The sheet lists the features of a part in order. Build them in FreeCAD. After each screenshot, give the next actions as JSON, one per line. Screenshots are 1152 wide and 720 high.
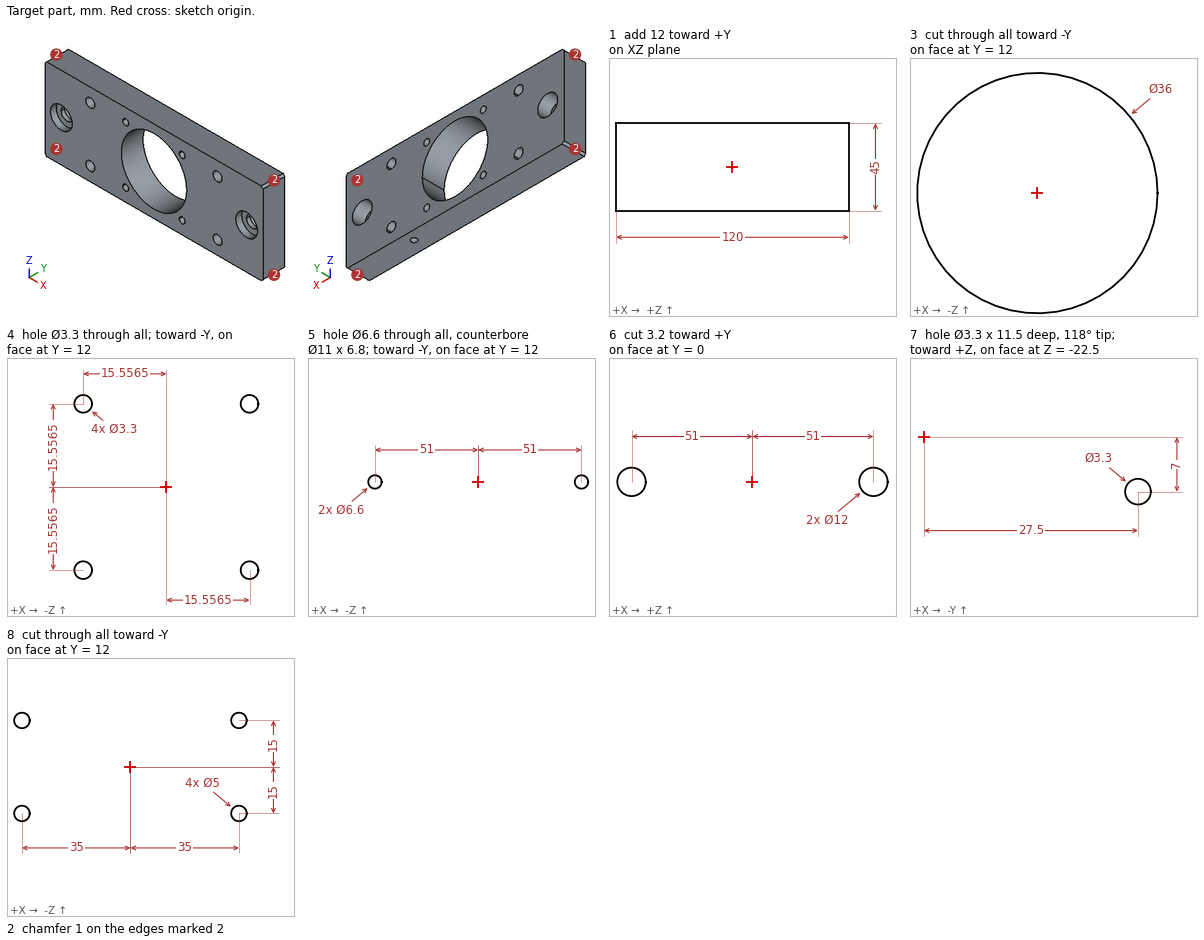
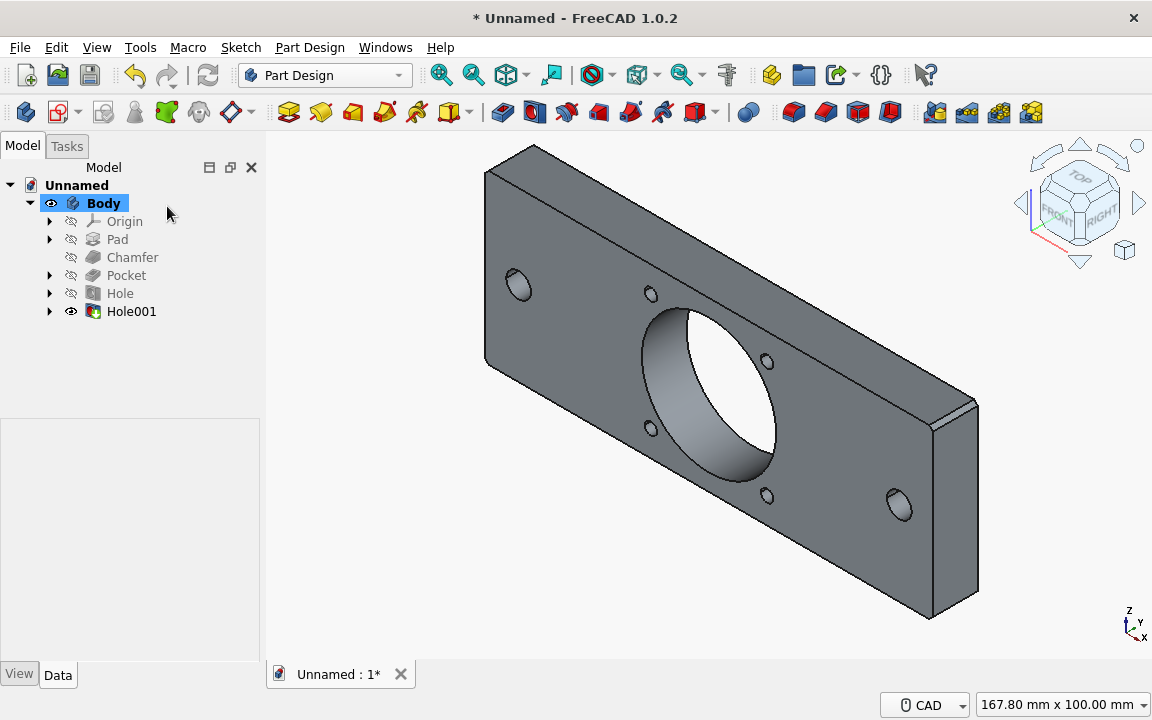
{"action": "left_click", "coordinate": [581, 292]}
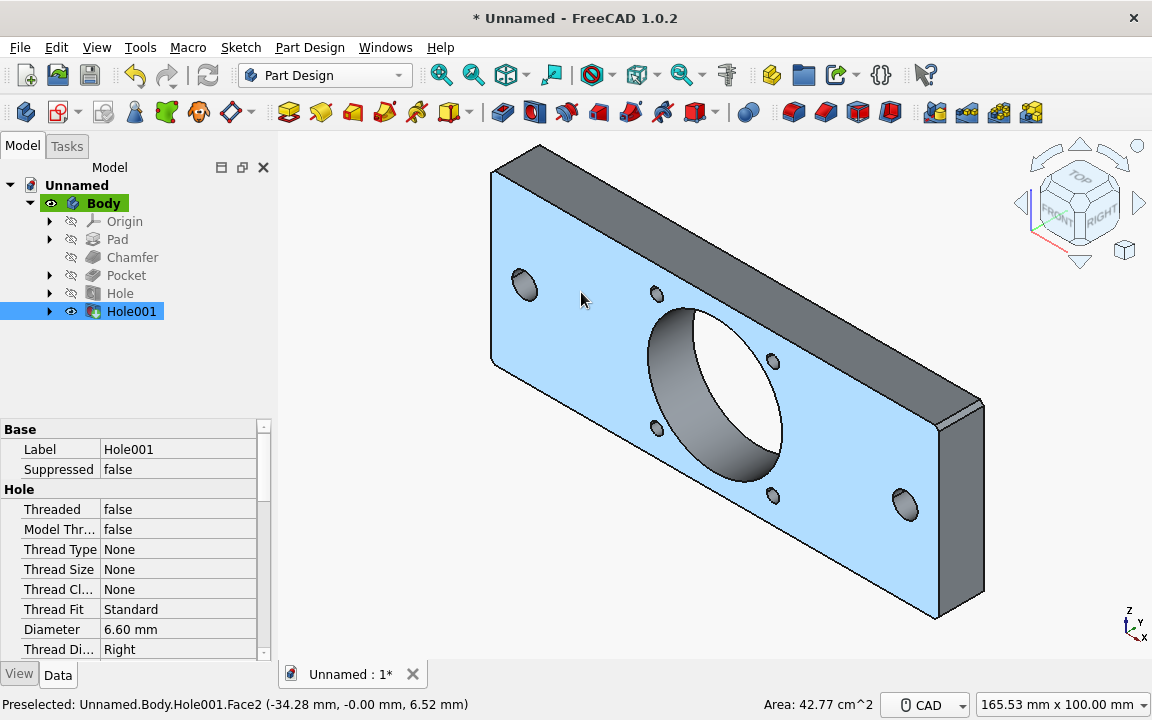
{"action": "left_click", "coordinate": [58, 112]}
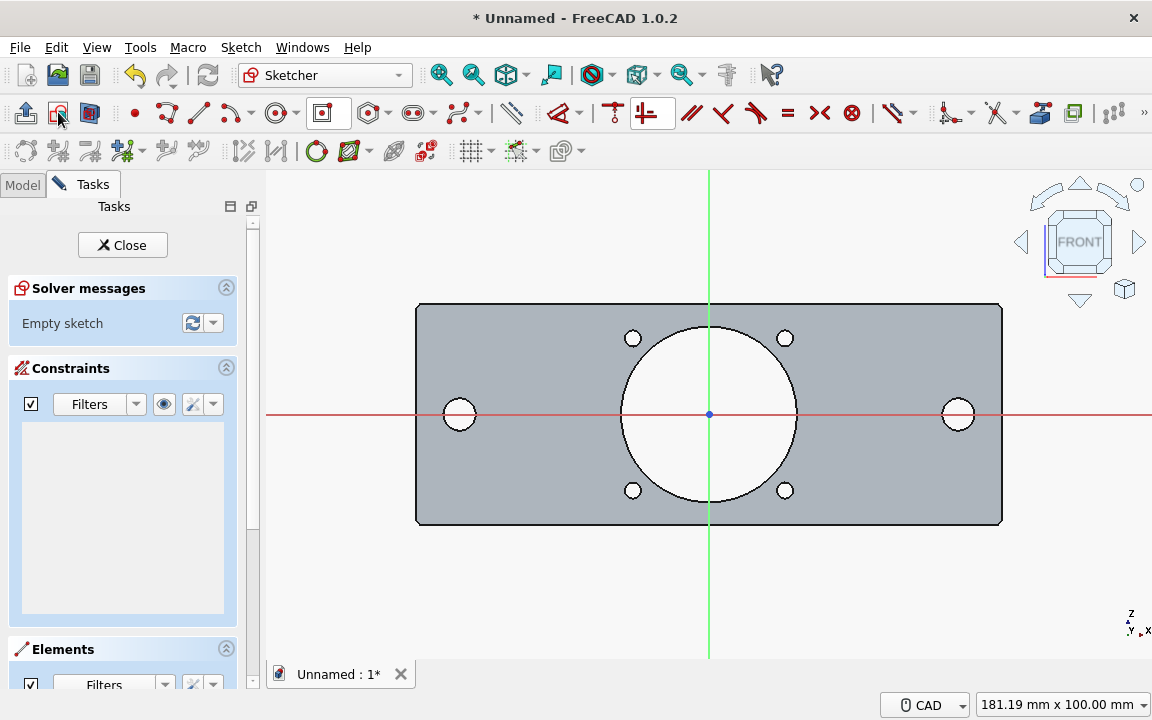
{"action": "scroll", "coordinate": [331, 415], "scroll_direction": "down", "scroll_amount": 1}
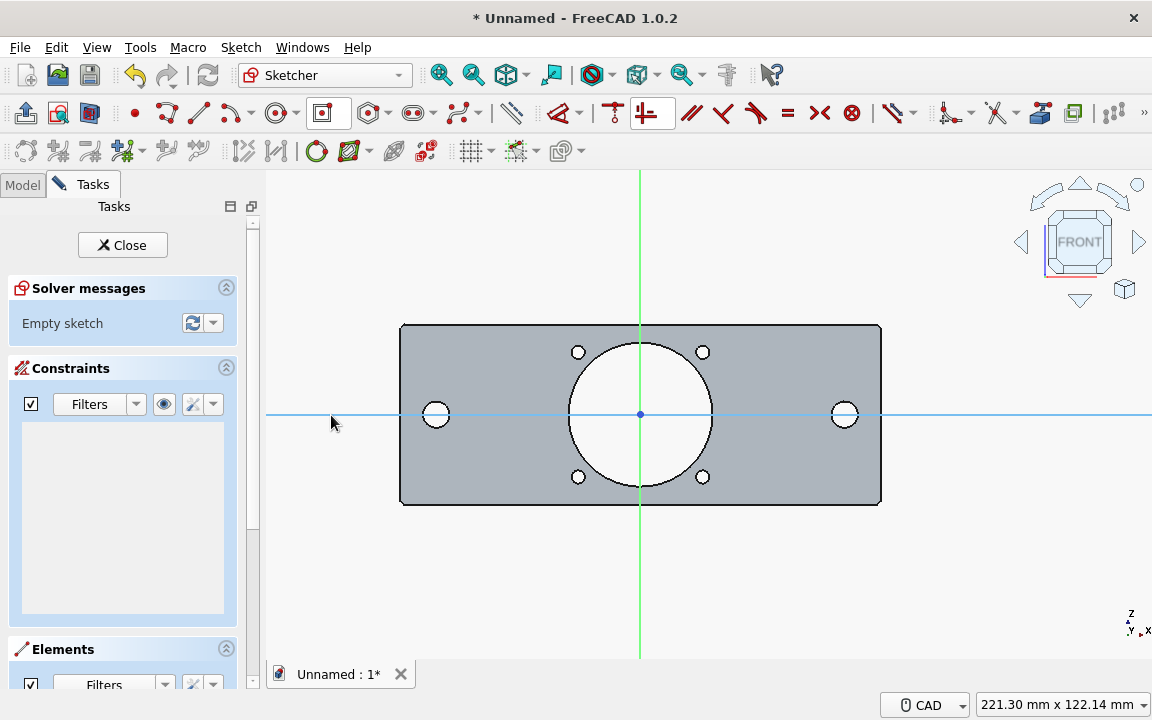
{"action": "left_click", "coordinate": [276, 114]}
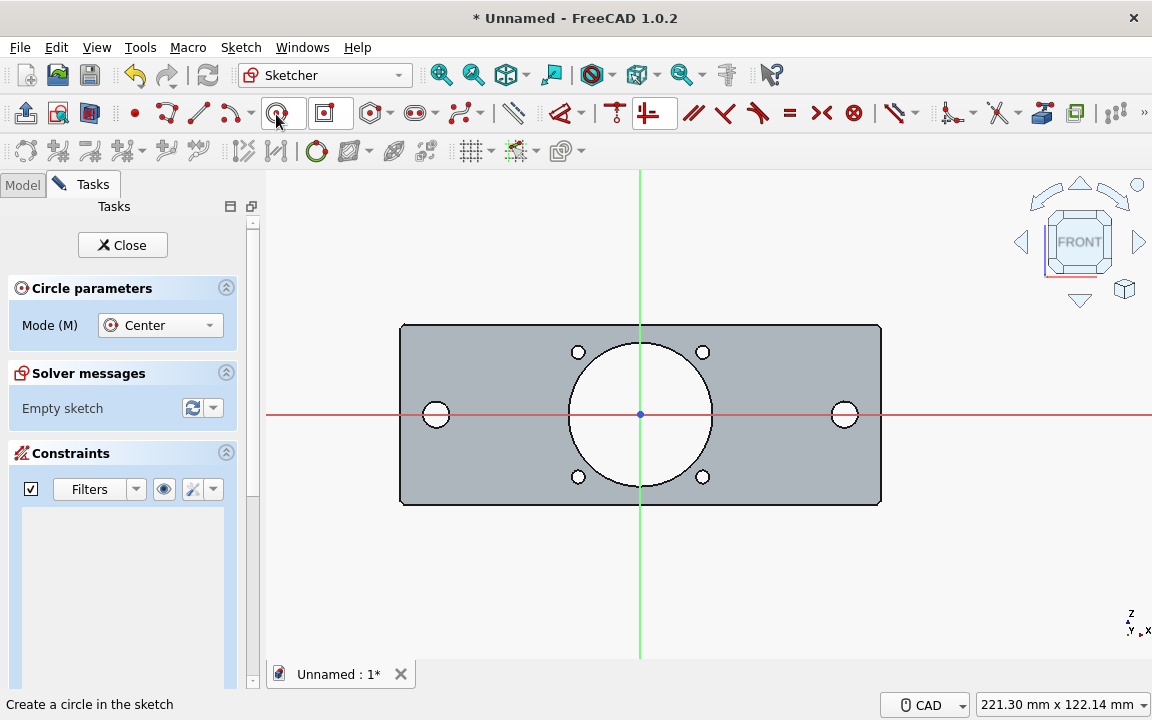
{"action": "left_click", "coordinate": [845, 415]}
{"action": "mouse_move", "coordinate": [862, 398]}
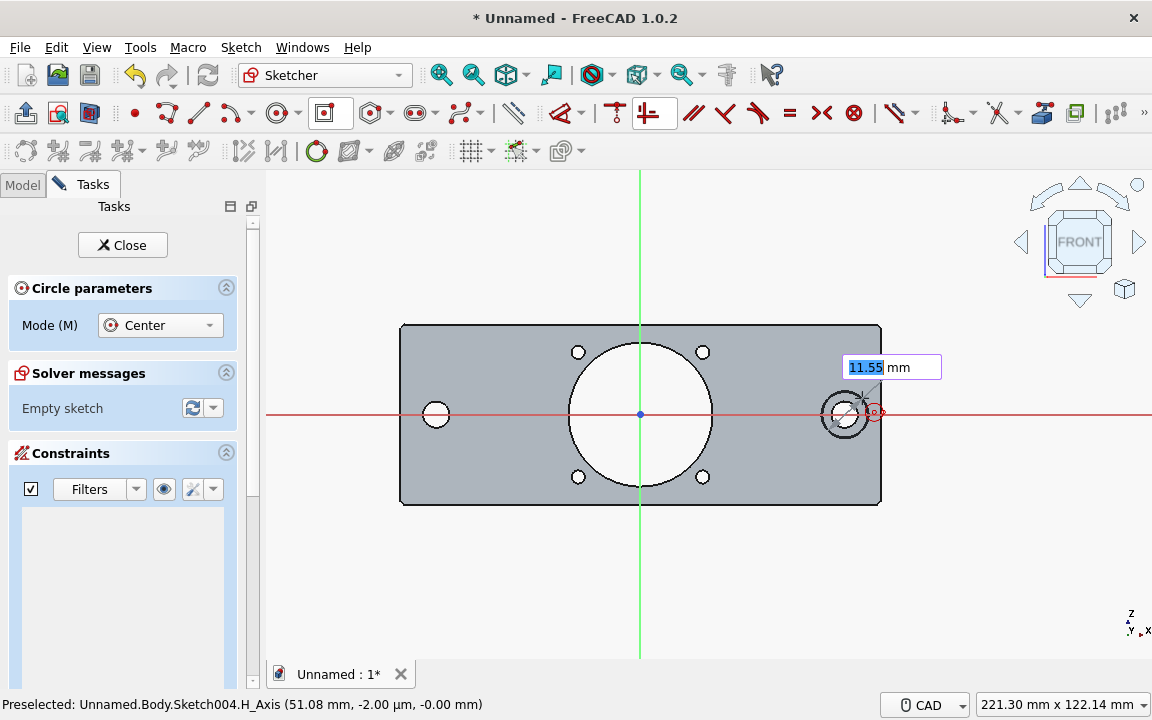
{"action": "type", "text": "12"}
{"action": "key", "text": "Return"}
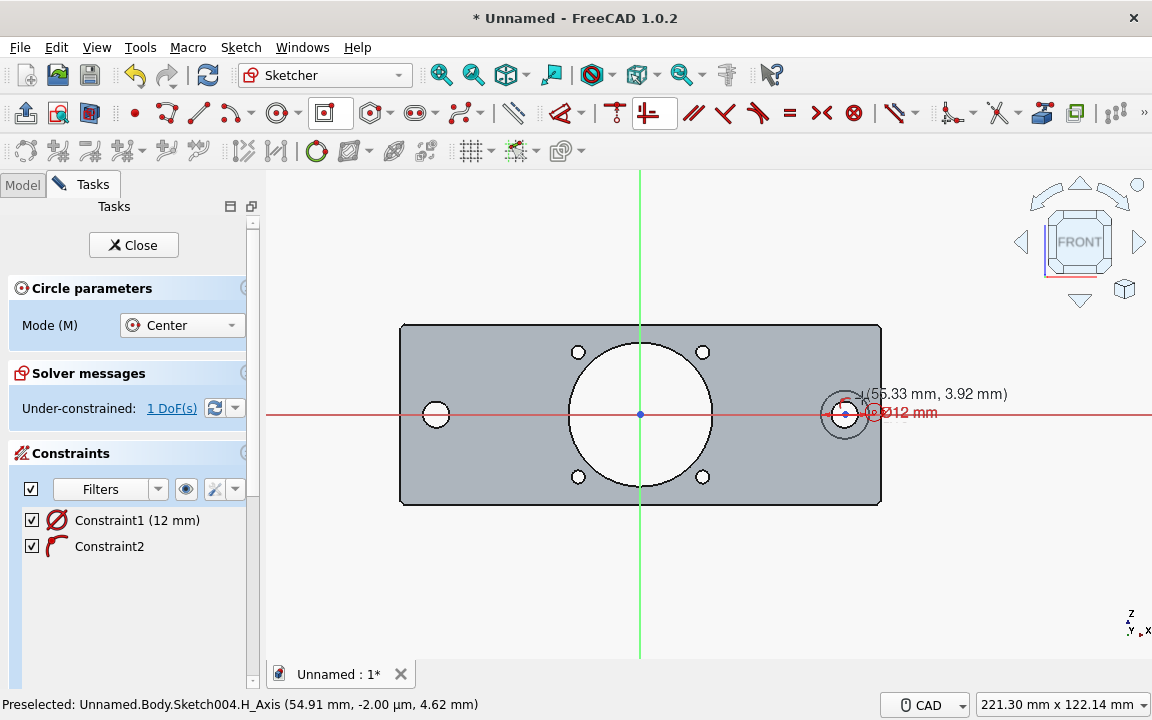
{"action": "left_click", "coordinate": [436, 415]}
{"action": "mouse_move", "coordinate": [453, 398]}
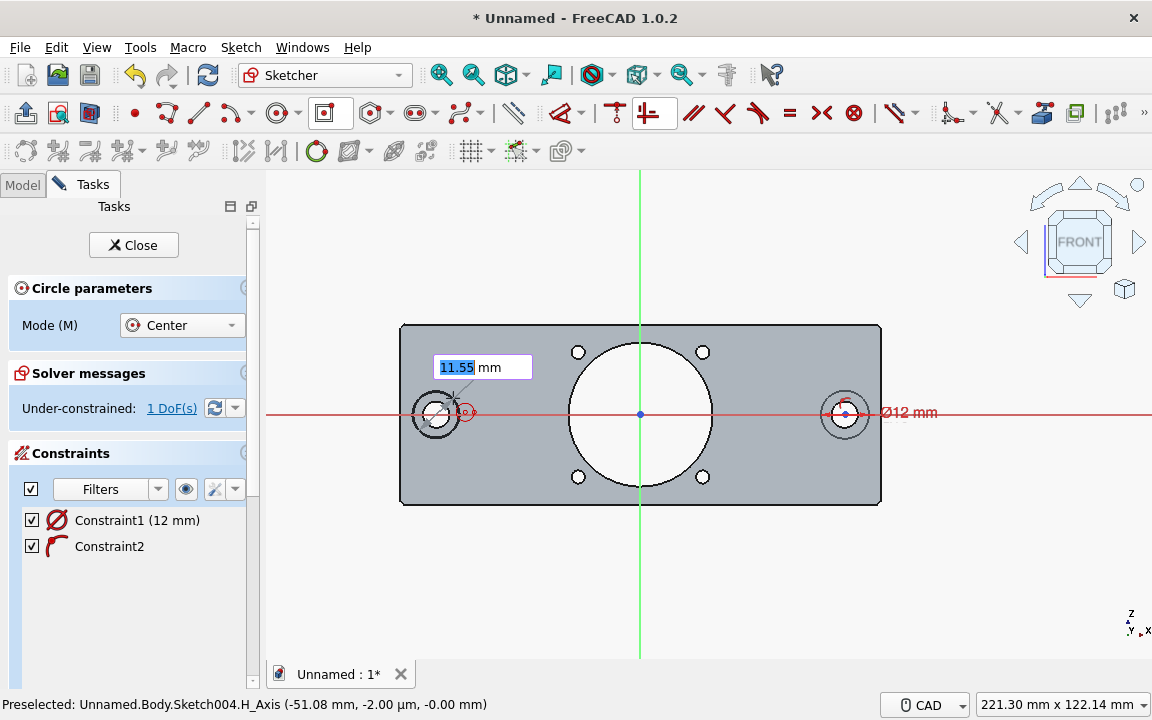
{"action": "type", "text": "12"}
{"action": "key", "text": "Return"}
{"action": "key", "text": "Escape"}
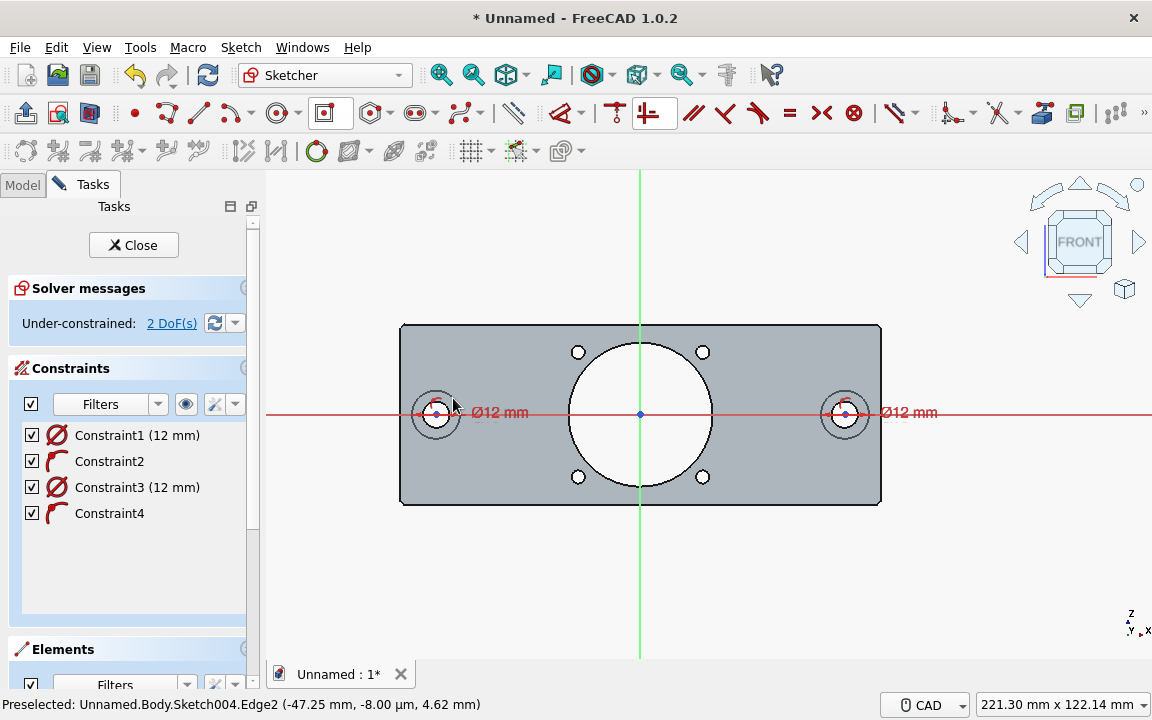
{"action": "left_click", "coordinate": [560, 114]}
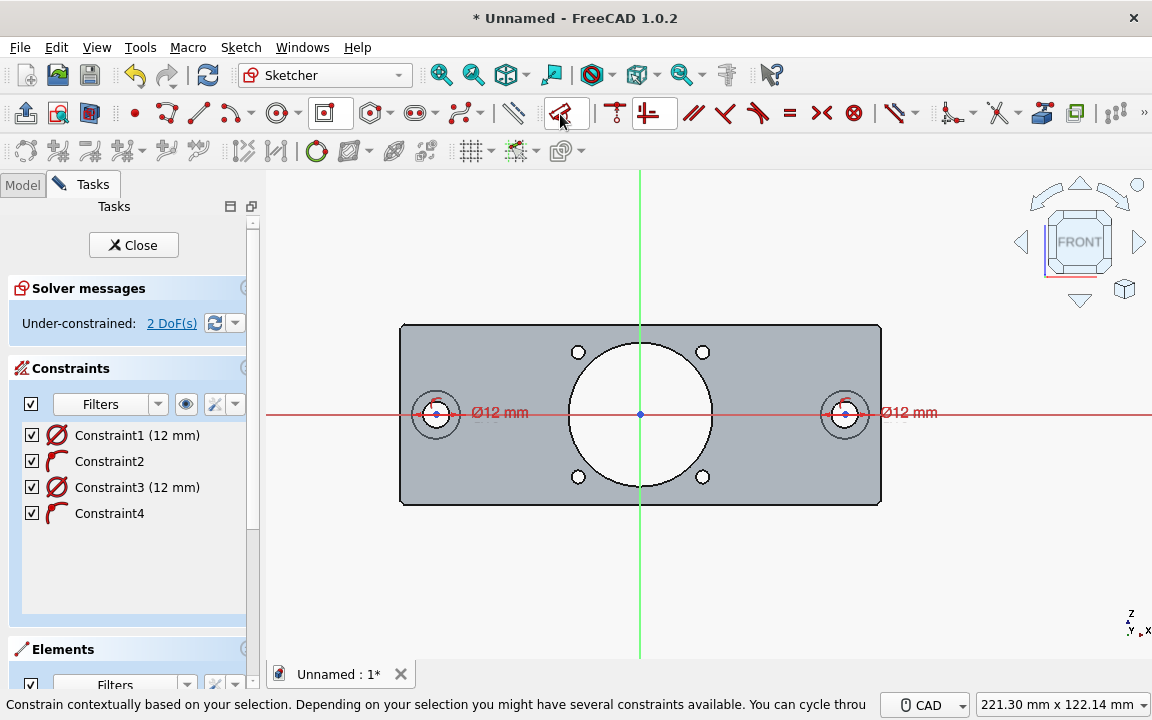
{"action": "left_click", "coordinate": [845, 415]}
{"action": "left_click", "coordinate": [743, 449]}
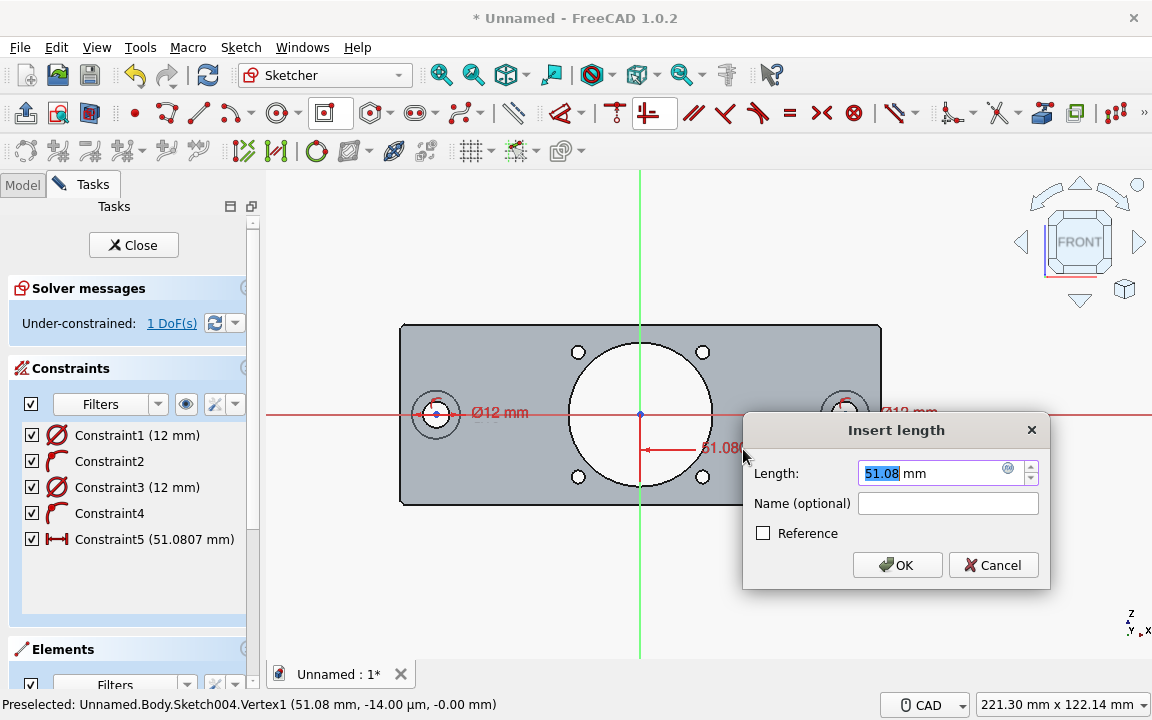
{"action": "type", "text": "51"}
{"action": "key", "text": "Return"}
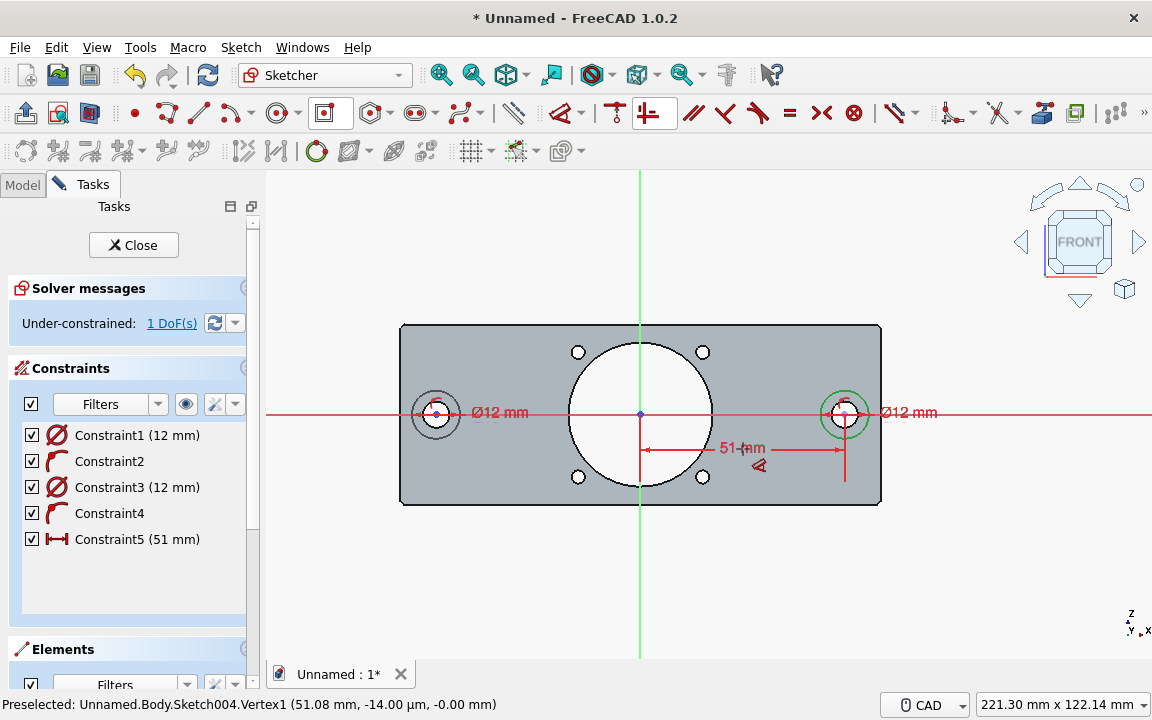
{"action": "left_click", "coordinate": [436, 415]}
{"action": "left_click", "coordinate": [538, 449]}